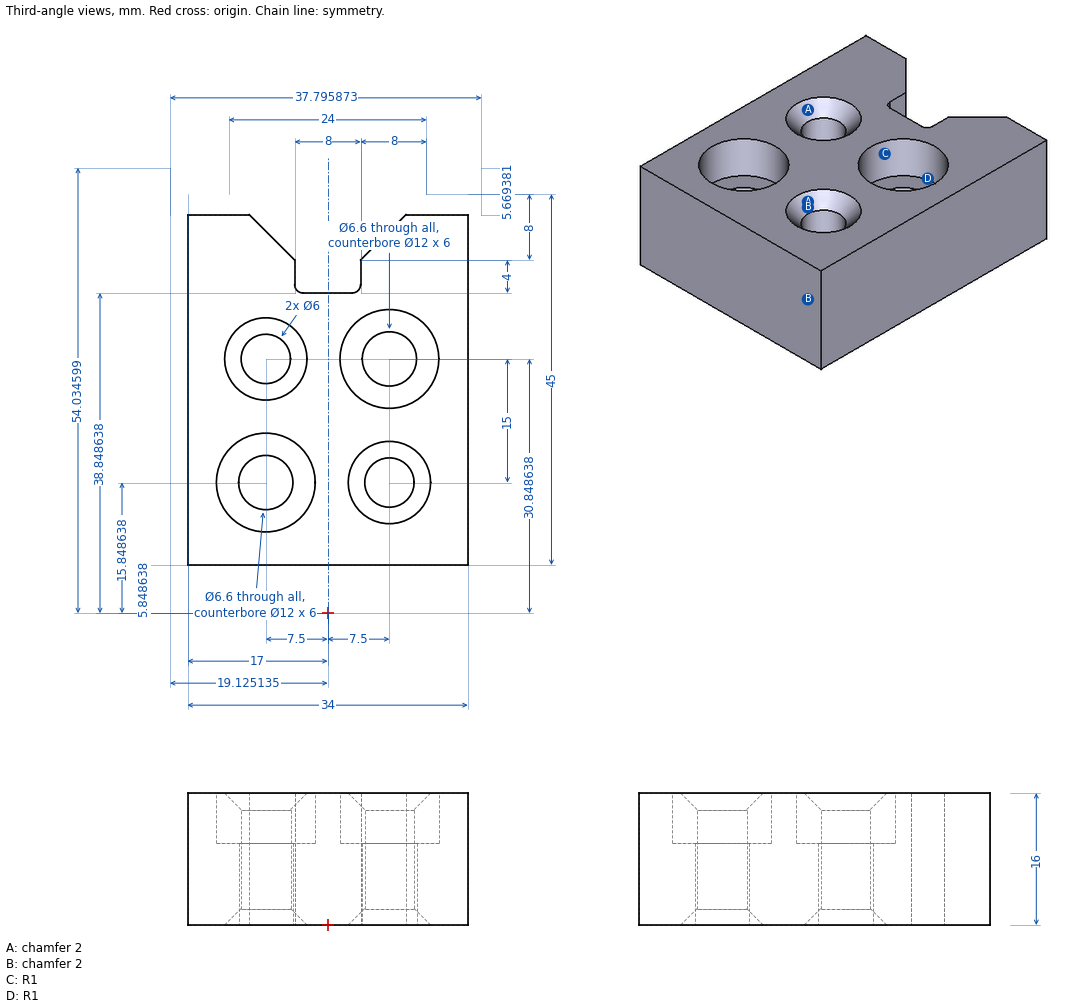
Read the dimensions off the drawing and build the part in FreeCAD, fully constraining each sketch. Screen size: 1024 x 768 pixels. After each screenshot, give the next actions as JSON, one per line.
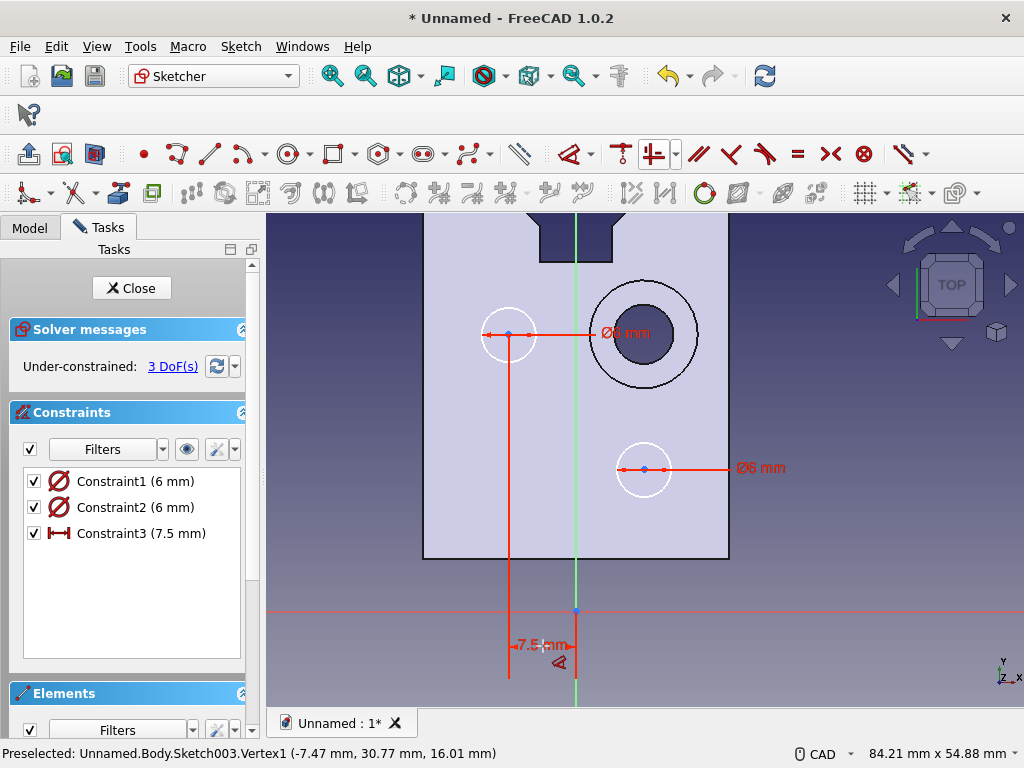
{"action": "left_click", "coordinate": [644, 470]}
{"action": "left_click", "coordinate": [626, 646]}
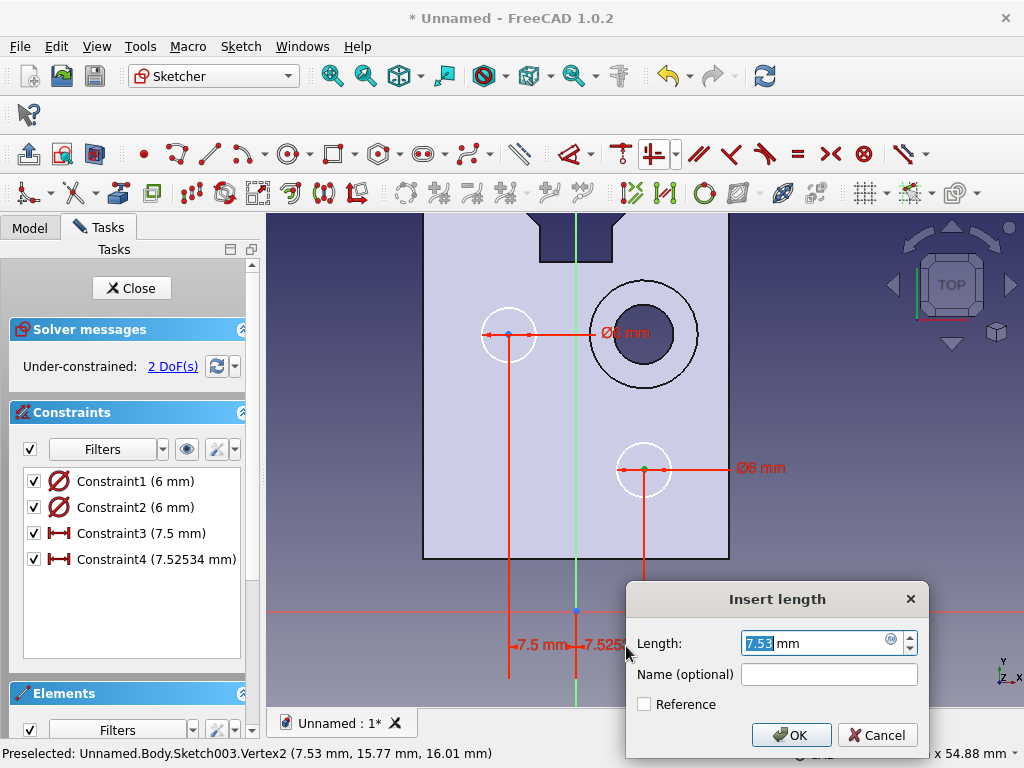
{"action": "type", "text": "7.5"}
{"action": "key", "text": "Return"}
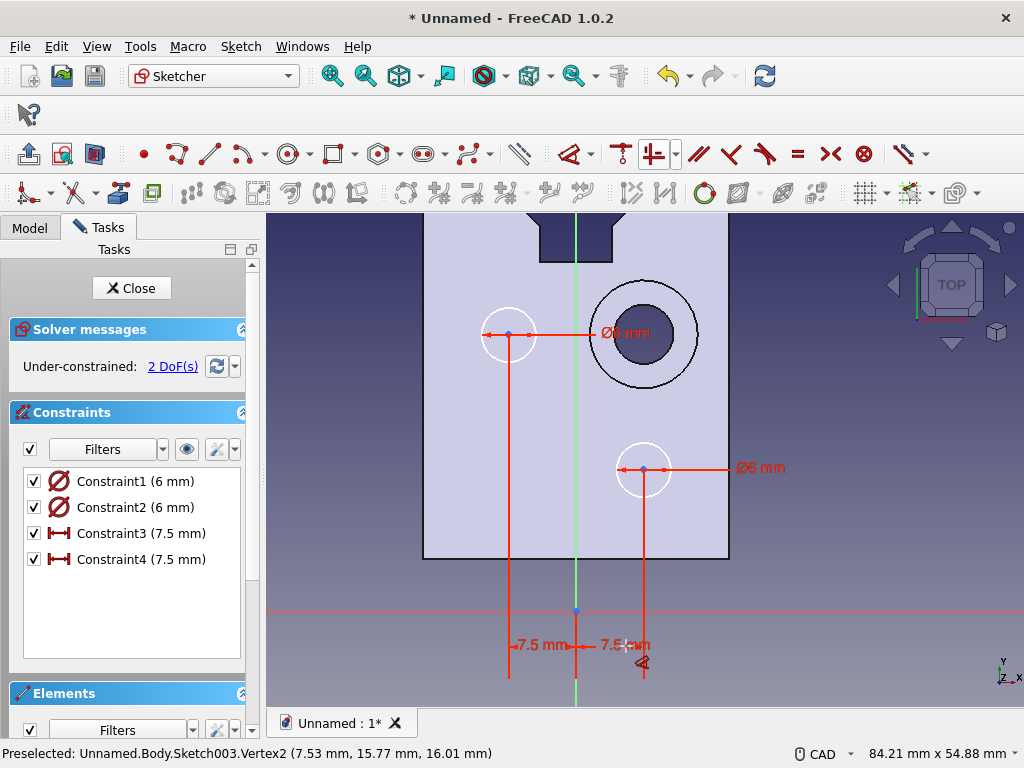
{"action": "left_click", "coordinate": [509, 335]}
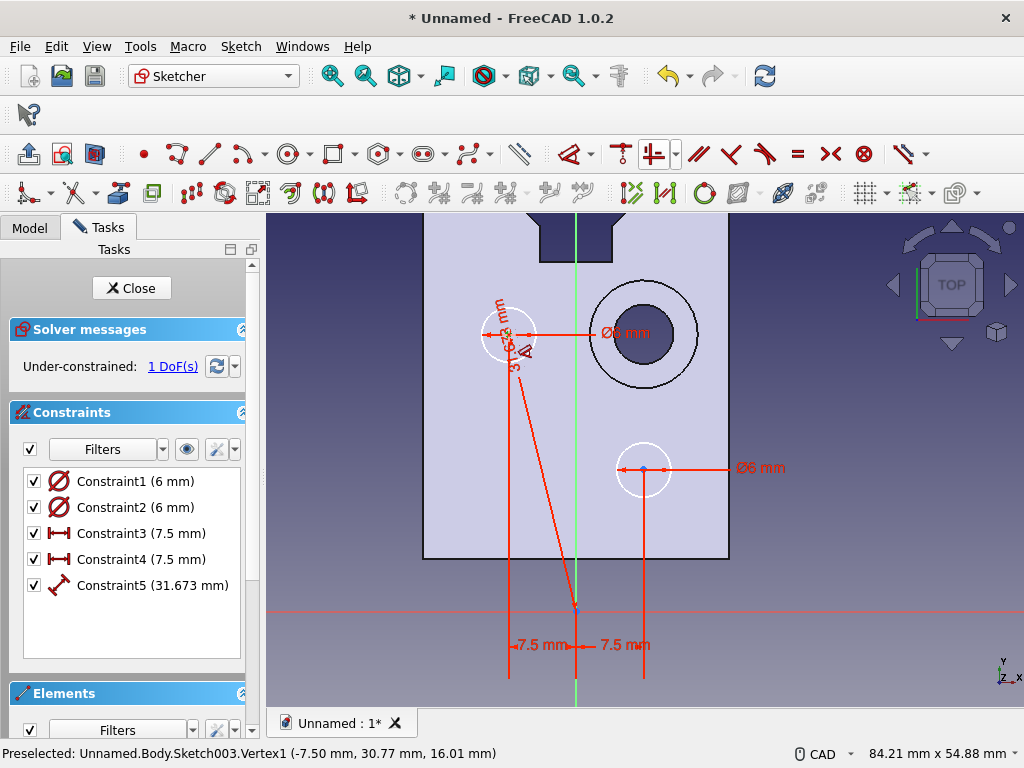
{"action": "left_click", "coordinate": [644, 470]}
{"action": "left_click", "coordinate": [678, 403]}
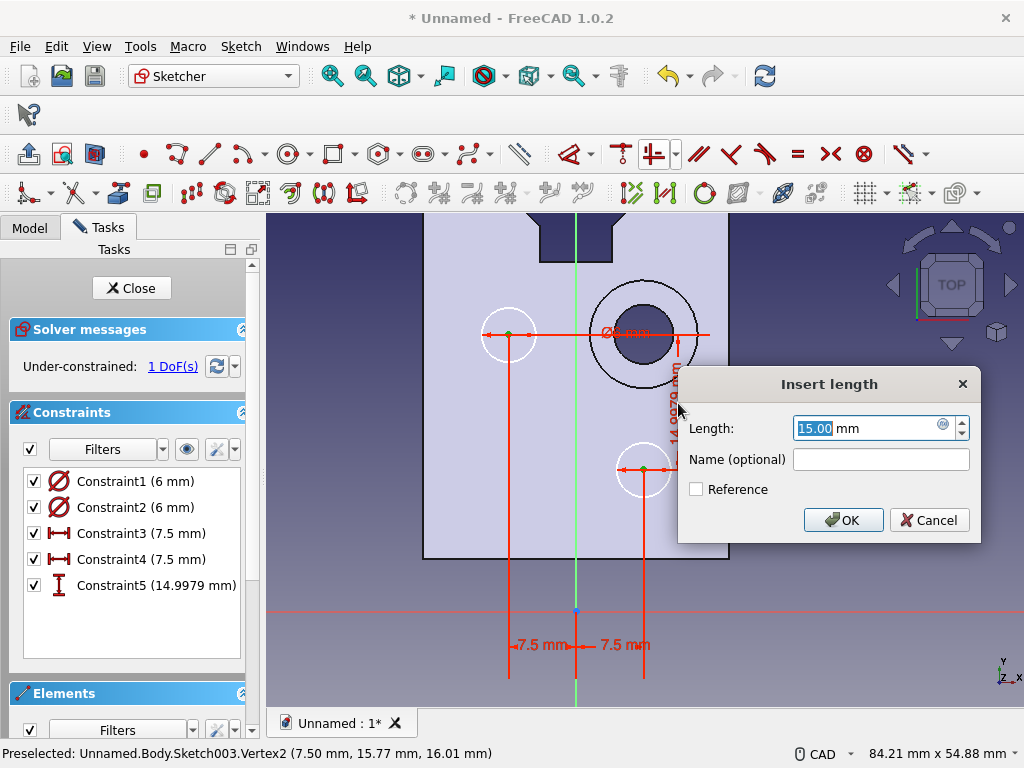
{"action": "type", "text": "15"}
{"action": "key", "text": "Return"}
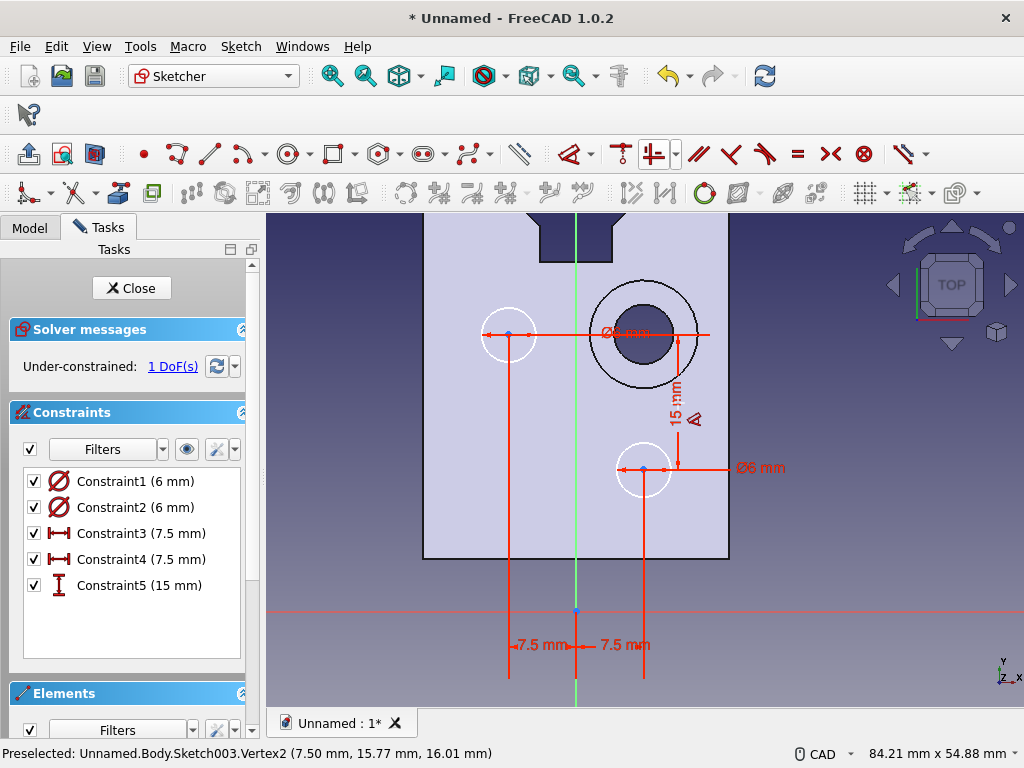
{"action": "left_click", "coordinate": [509, 335]}
{"action": "left_click", "coordinate": [475, 473]}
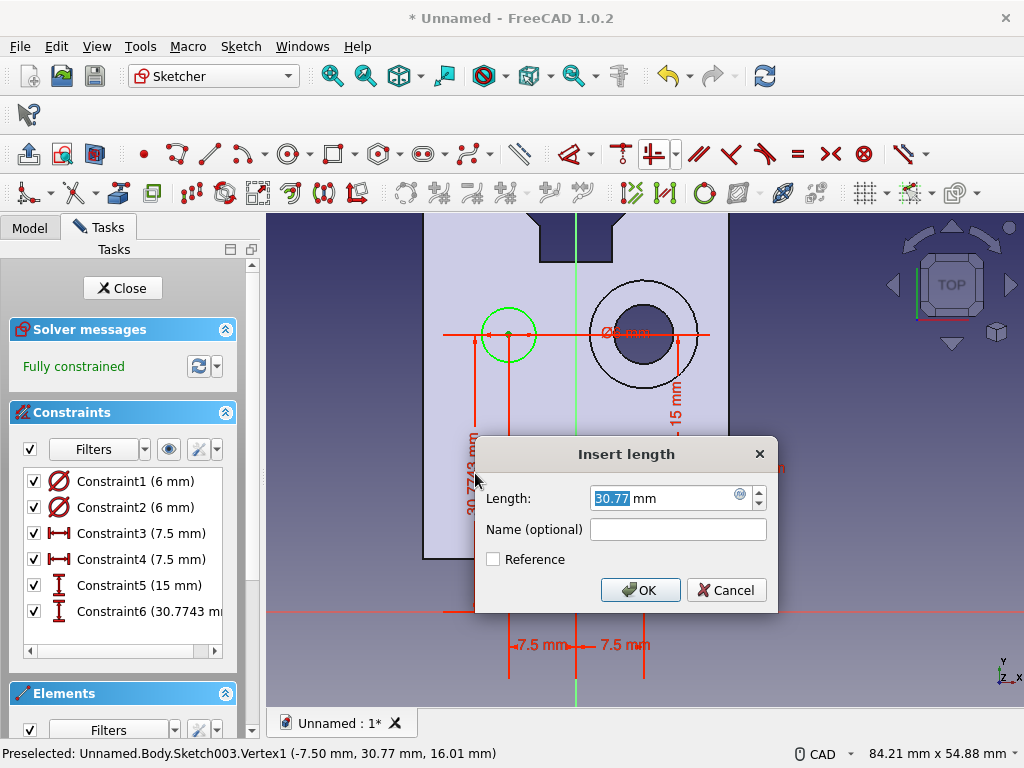
{"action": "type", "text": "30.848638"}
{"action": "key", "text": "Return"}
{"action": "key", "text": "Escape"}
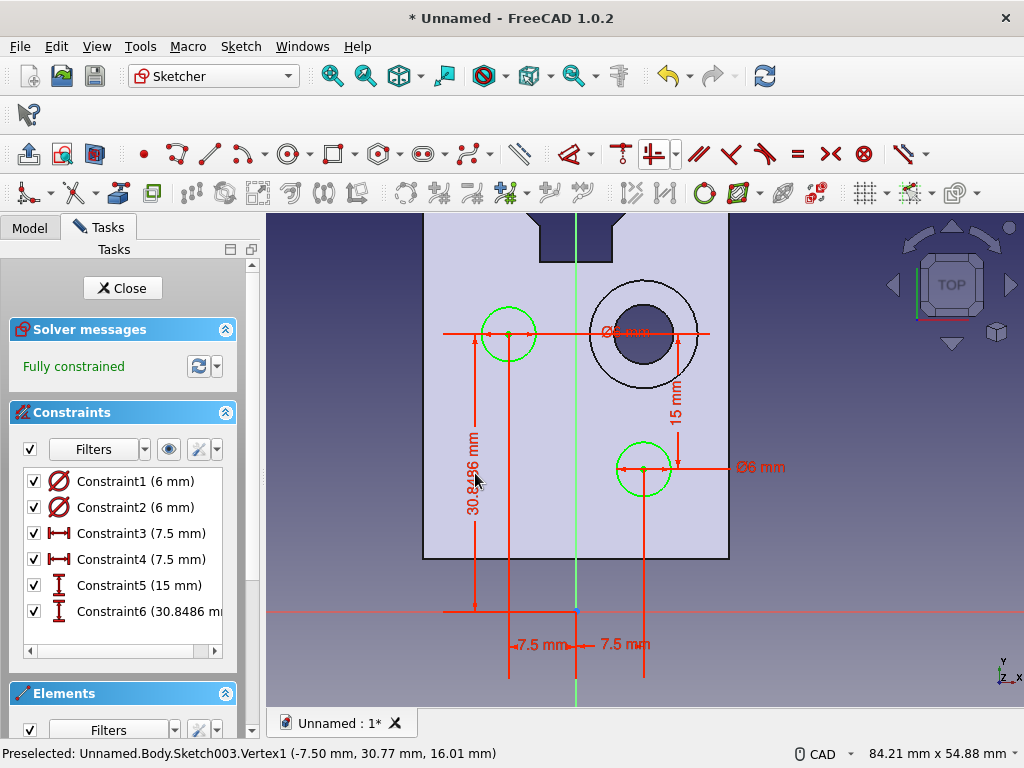
{"action": "left_click", "coordinate": [123, 288]}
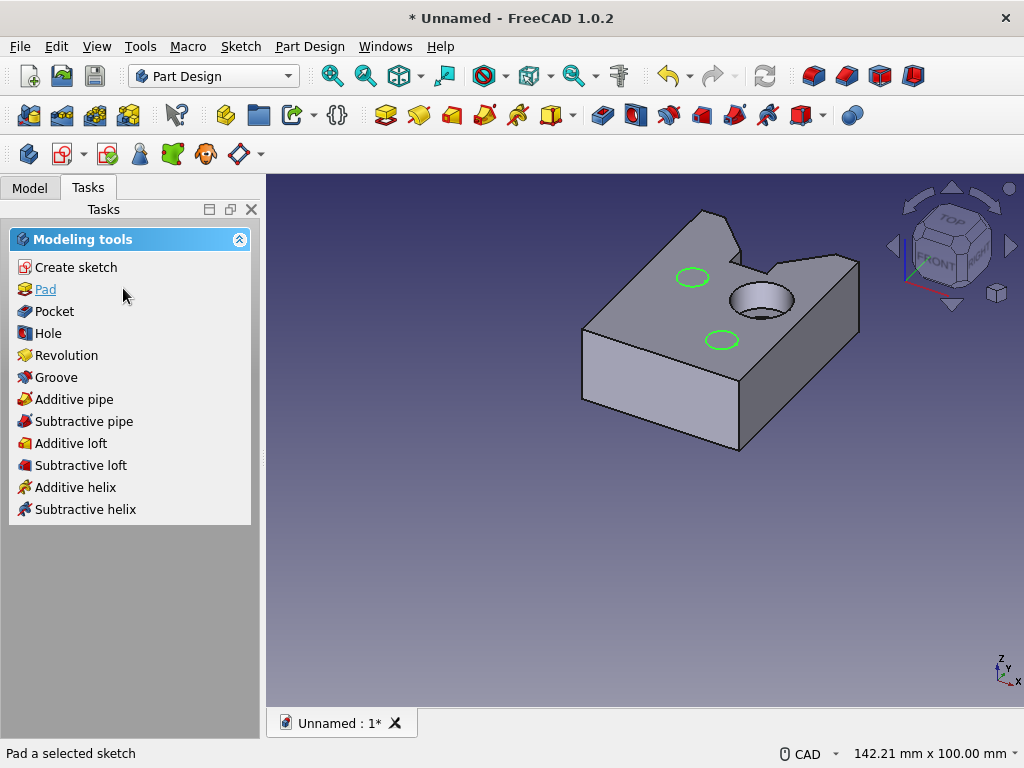
{"action": "left_click", "coordinate": [603, 116]}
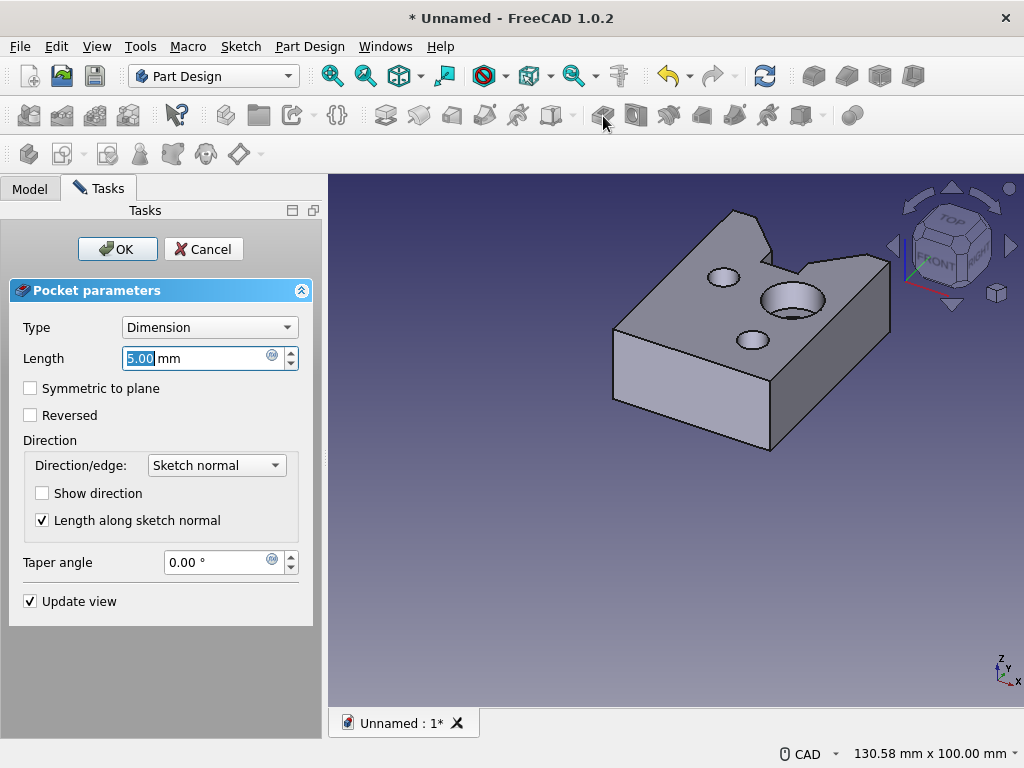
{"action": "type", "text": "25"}
{"action": "key", "text": "Tab"}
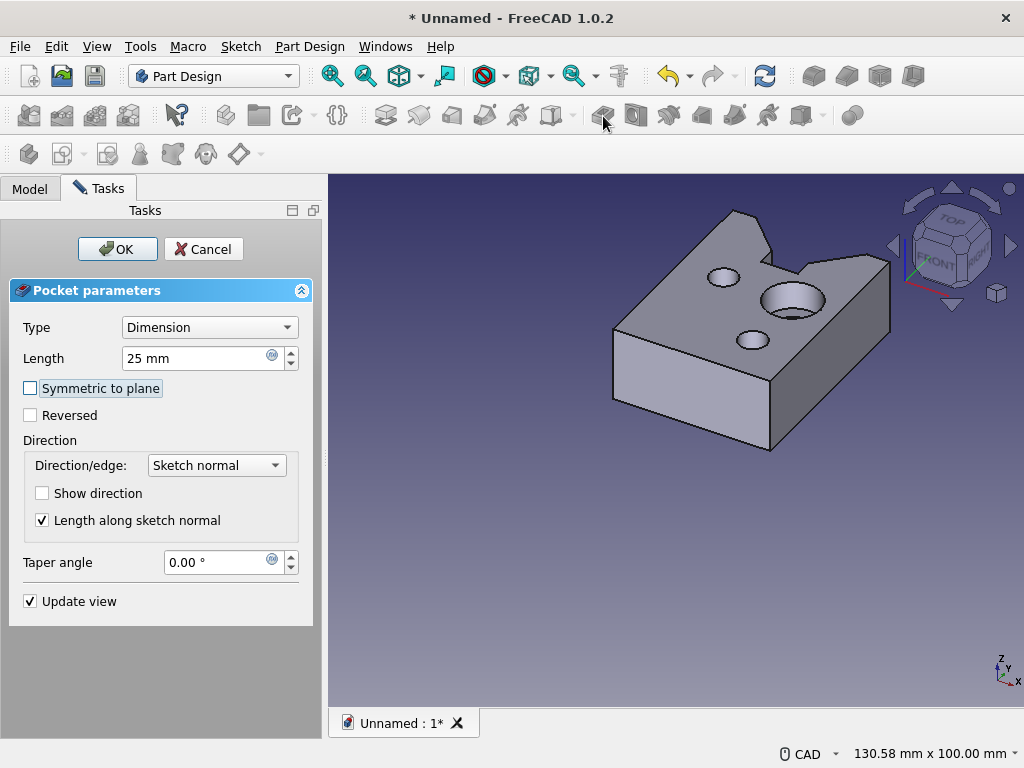
{"action": "left_click", "coordinate": [118, 249]}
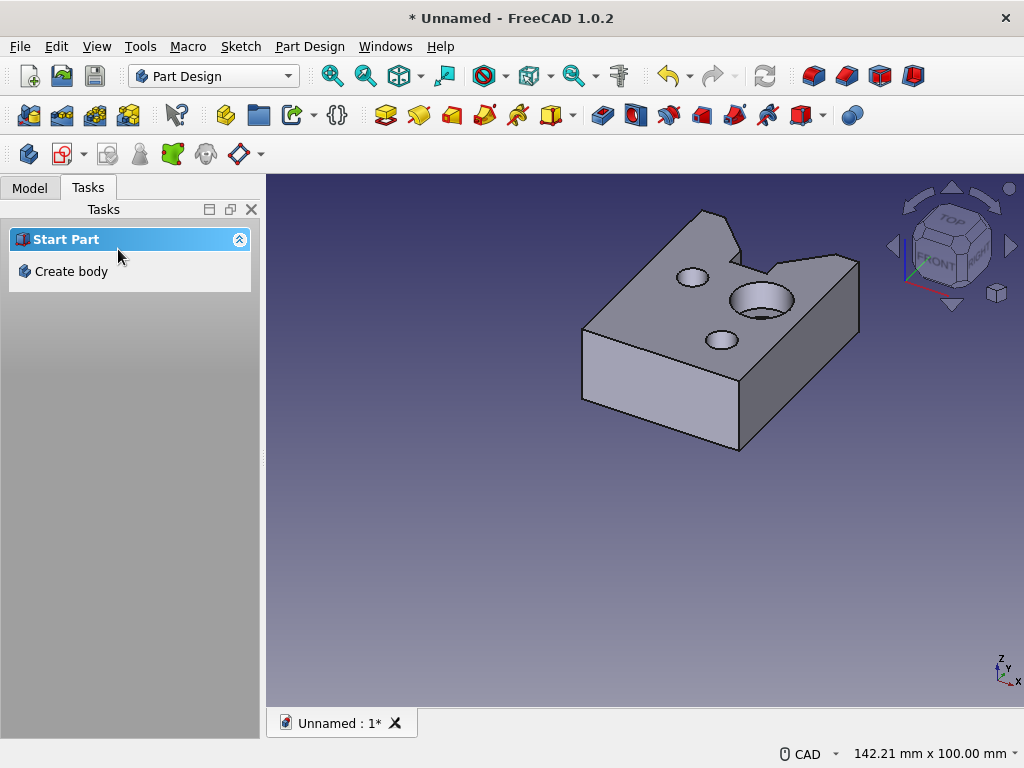
{"action": "left_click", "coordinate": [679, 272]}